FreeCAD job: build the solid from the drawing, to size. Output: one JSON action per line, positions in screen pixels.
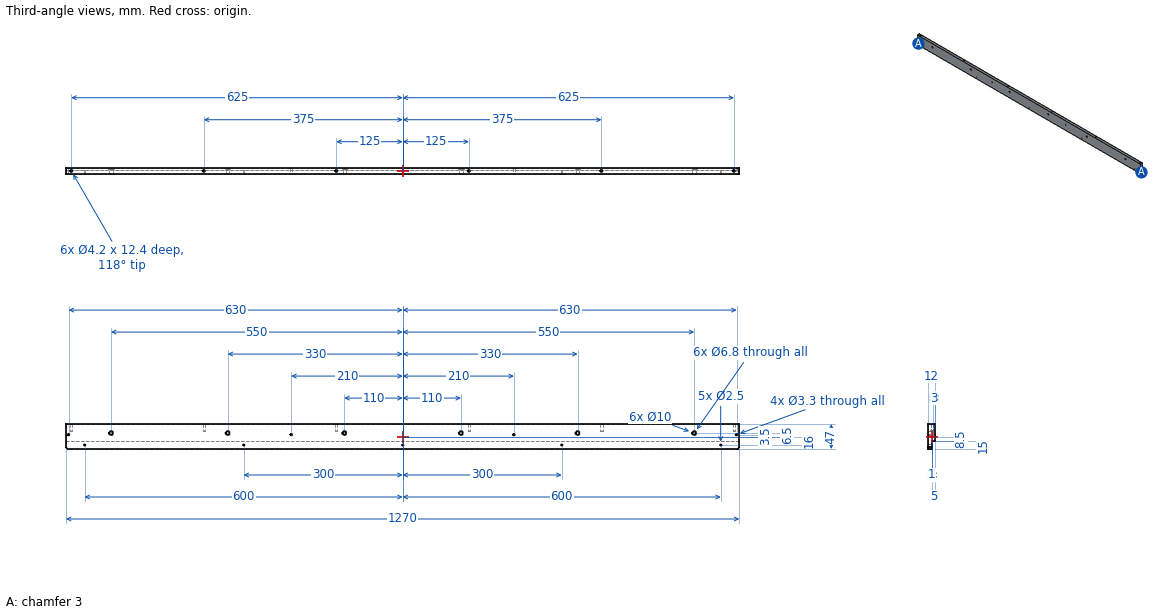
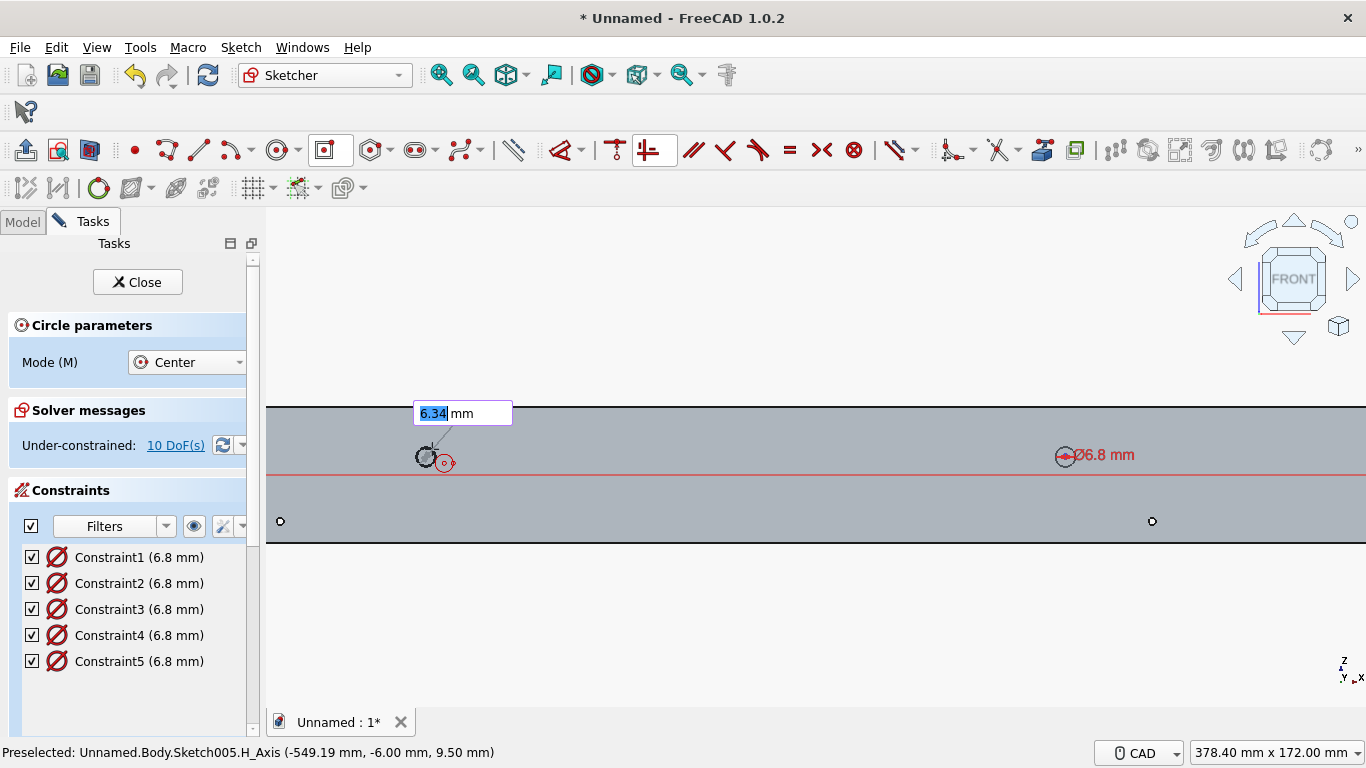
{"action": "type", "text": "6.8"}
{"action": "key", "text": "Return"}
{"action": "key", "text": "Escape"}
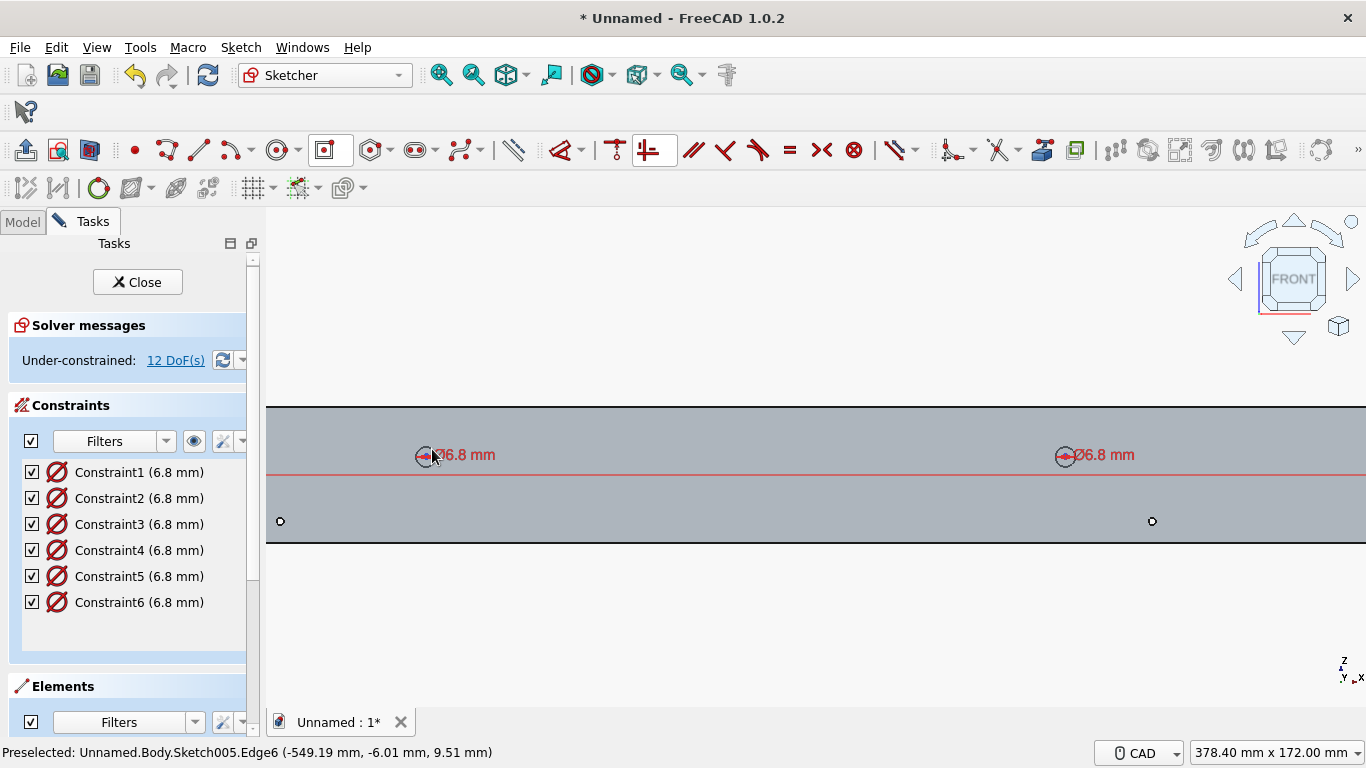
{"action": "scroll", "coordinate": [425, 456], "scroll_direction": "down", "scroll_amount": 8}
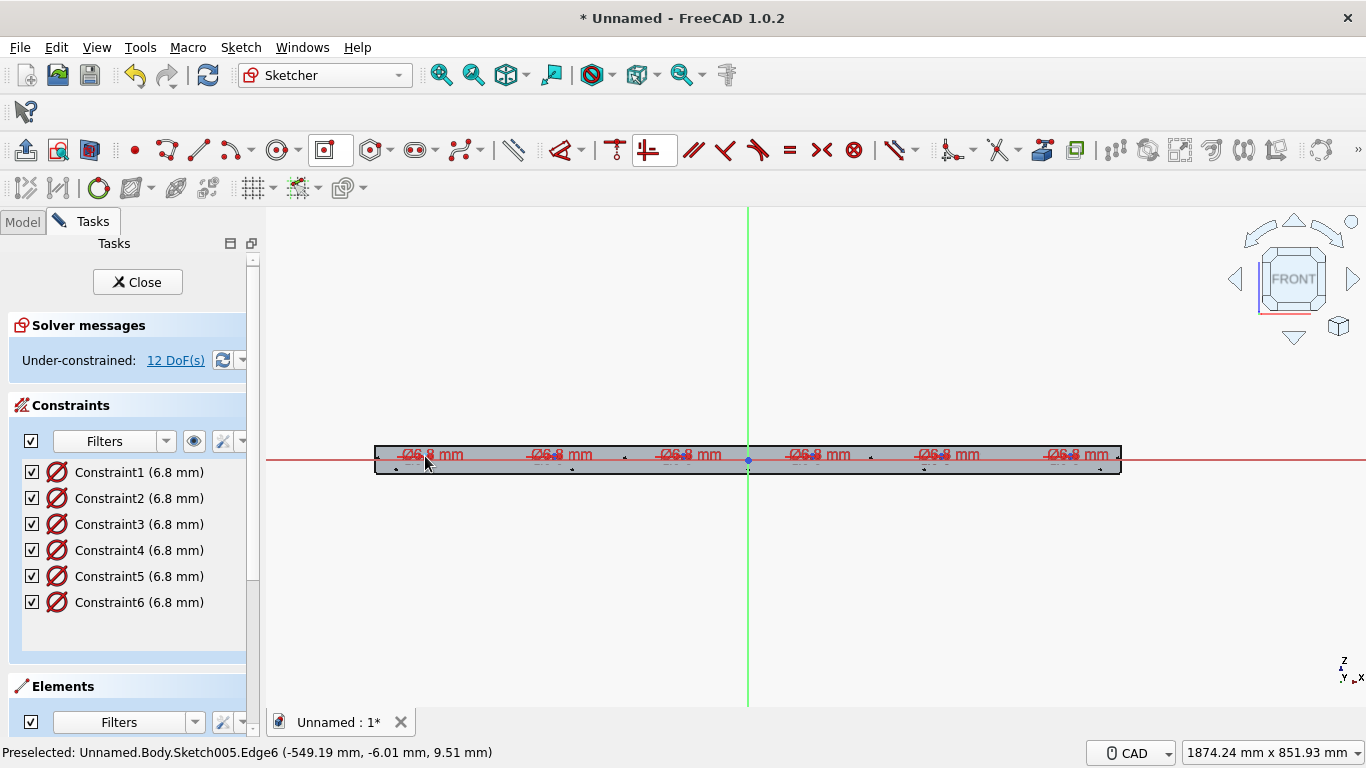
{"action": "left_click", "coordinate": [1071, 457]}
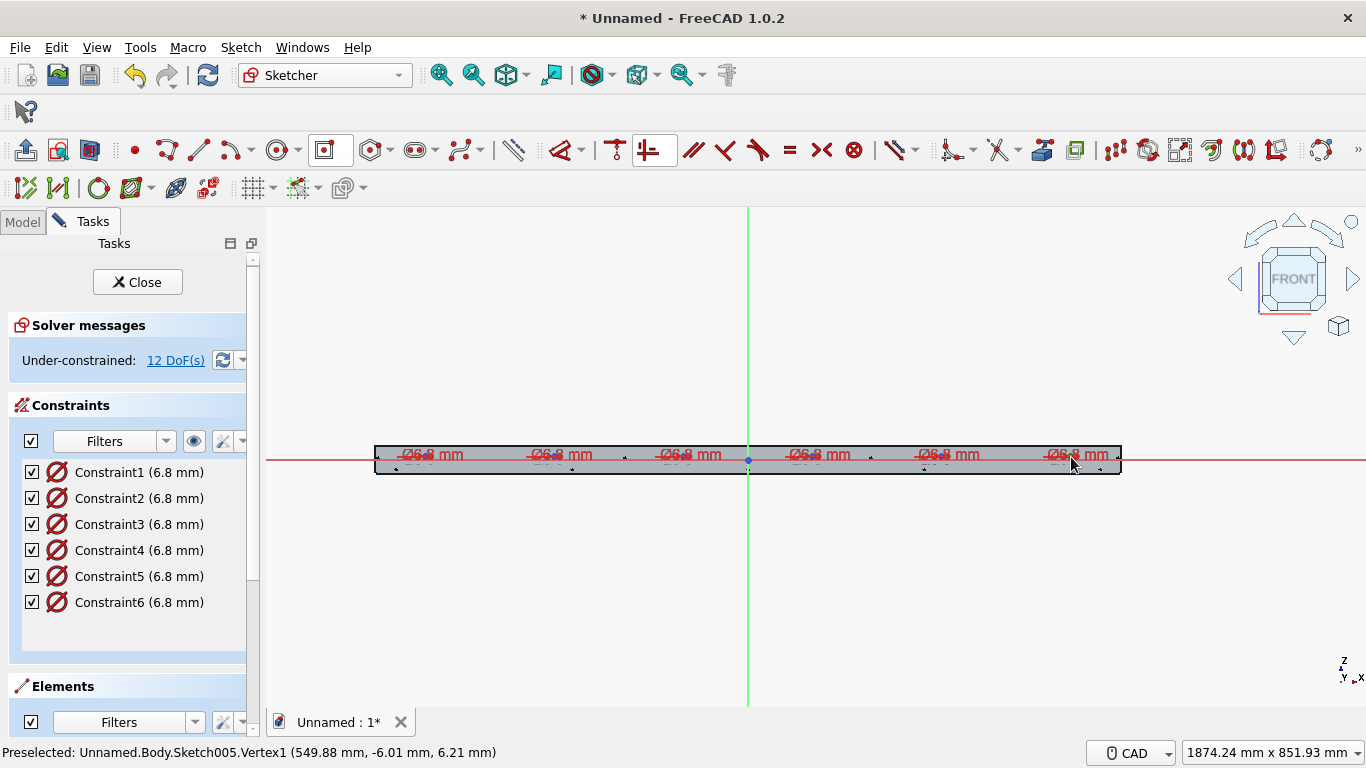
{"action": "left_click", "coordinate": [942, 457]}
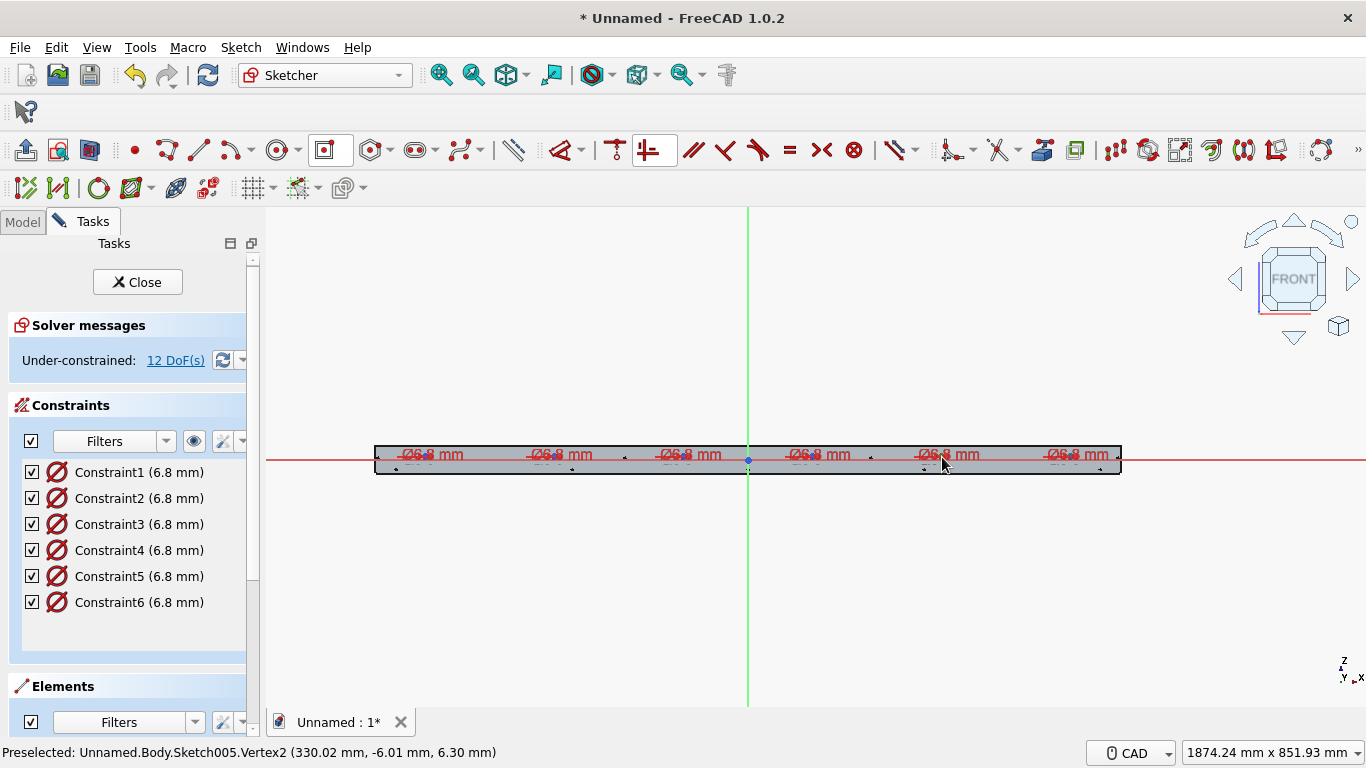
{"action": "key", "text": "h"}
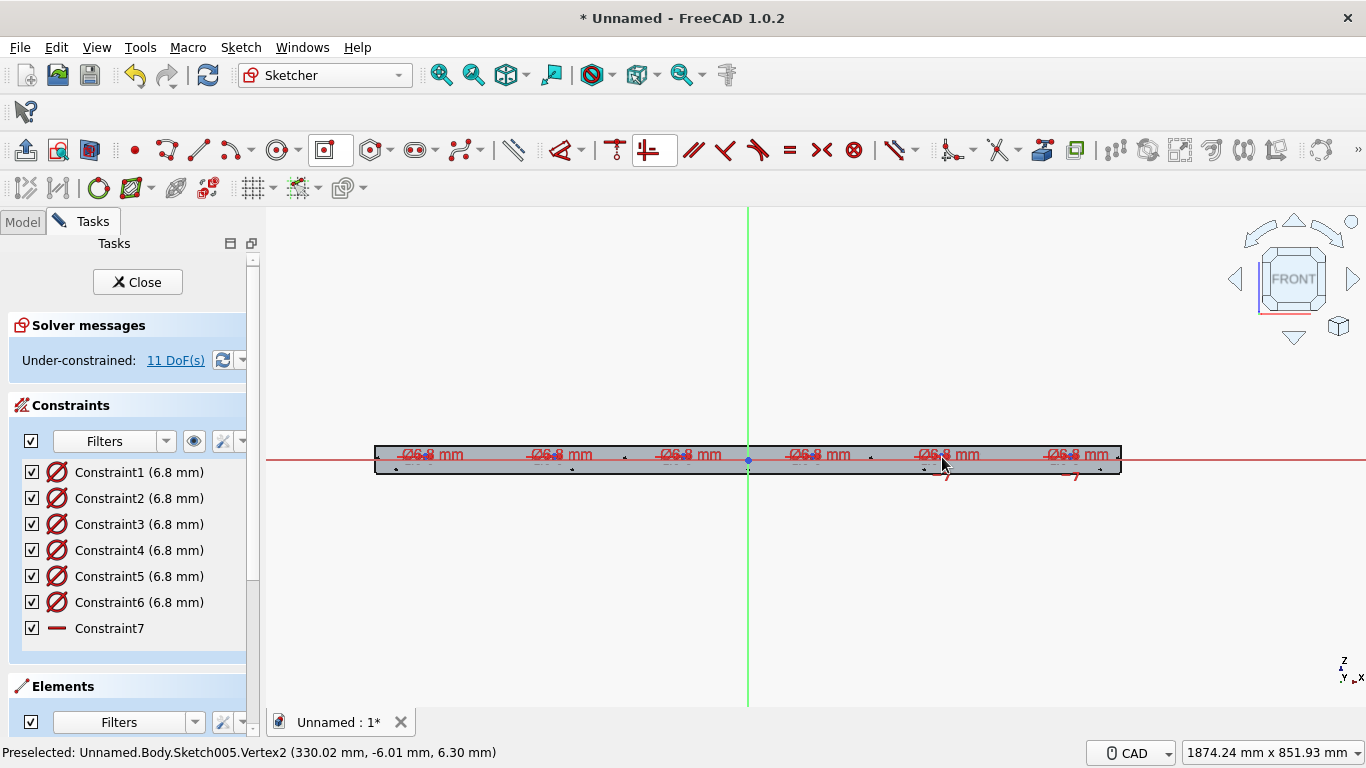
{"action": "left_click", "coordinate": [942, 457]}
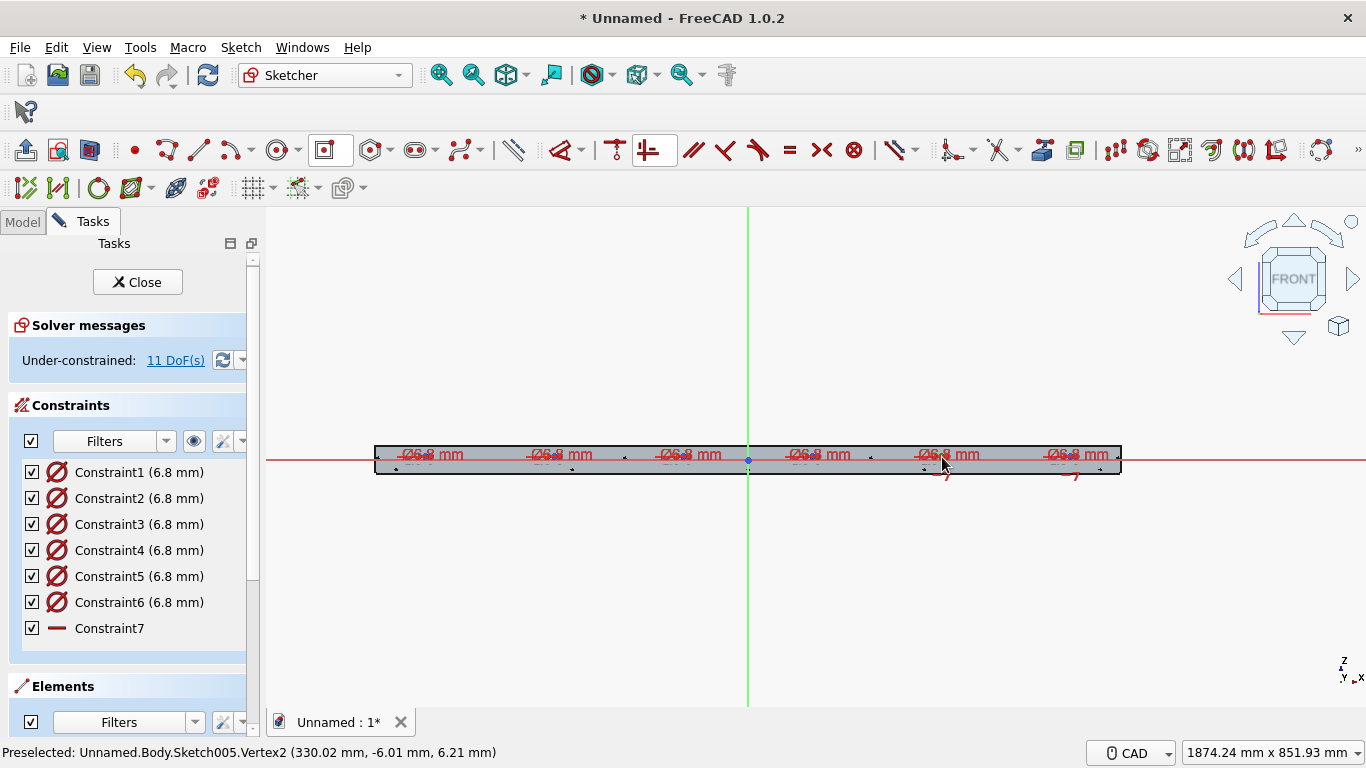
{"action": "left_click", "coordinate": [813, 457]}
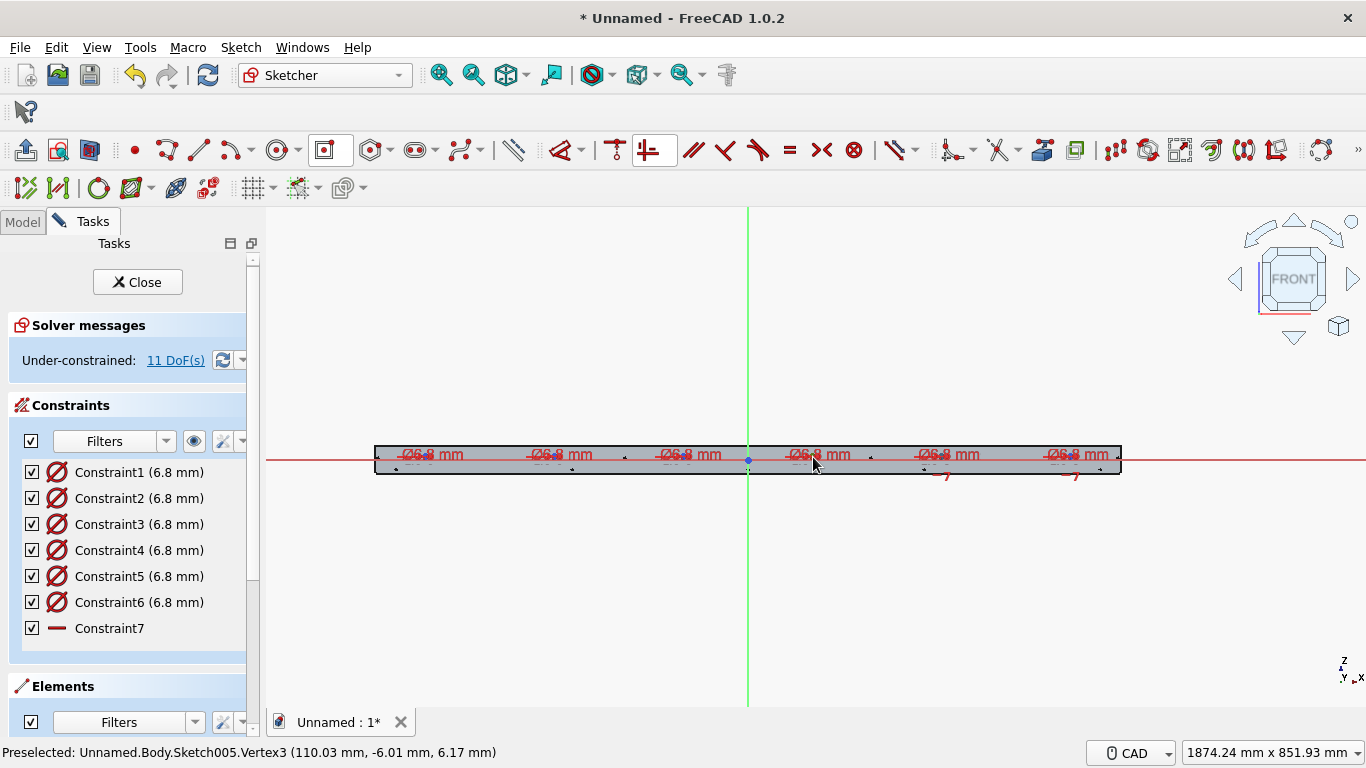
{"action": "left_click", "coordinate": [672, 150]}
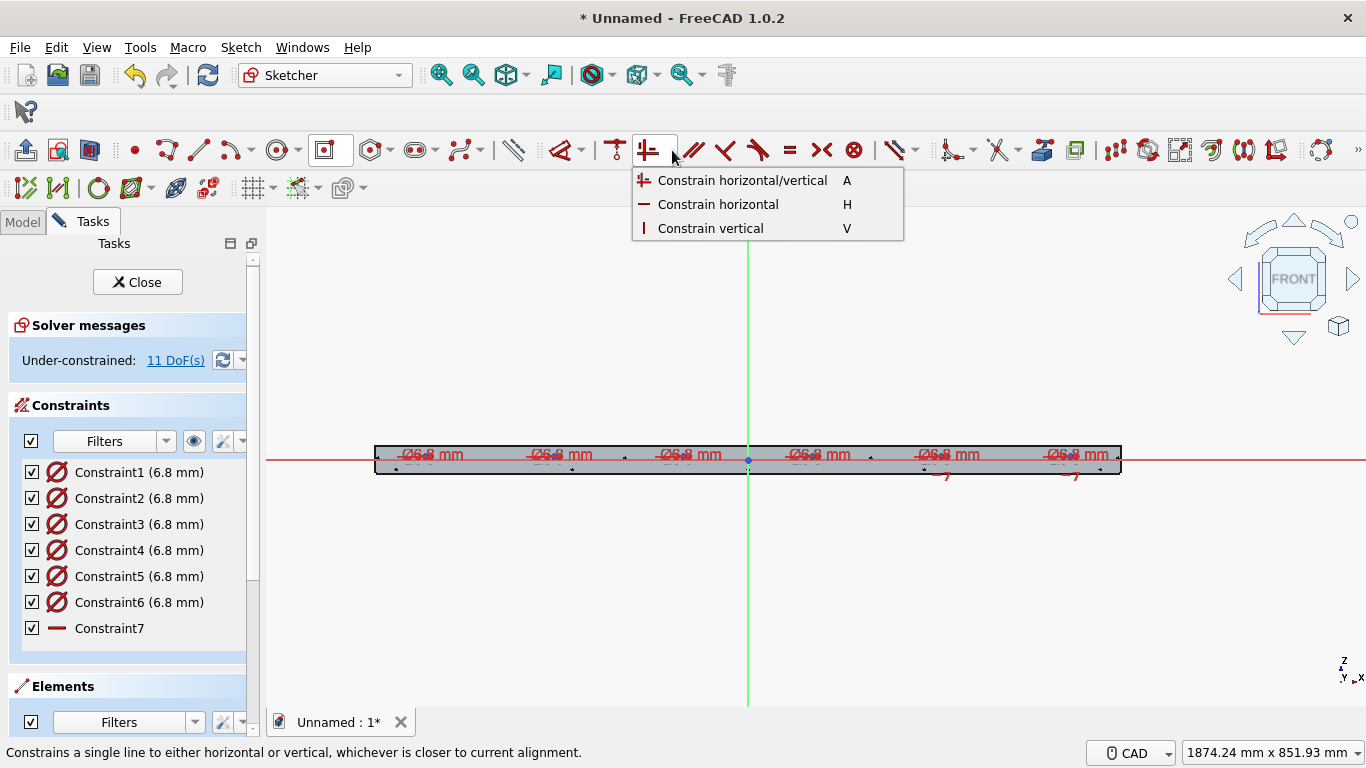
{"action": "left_click", "coordinate": [768, 204]}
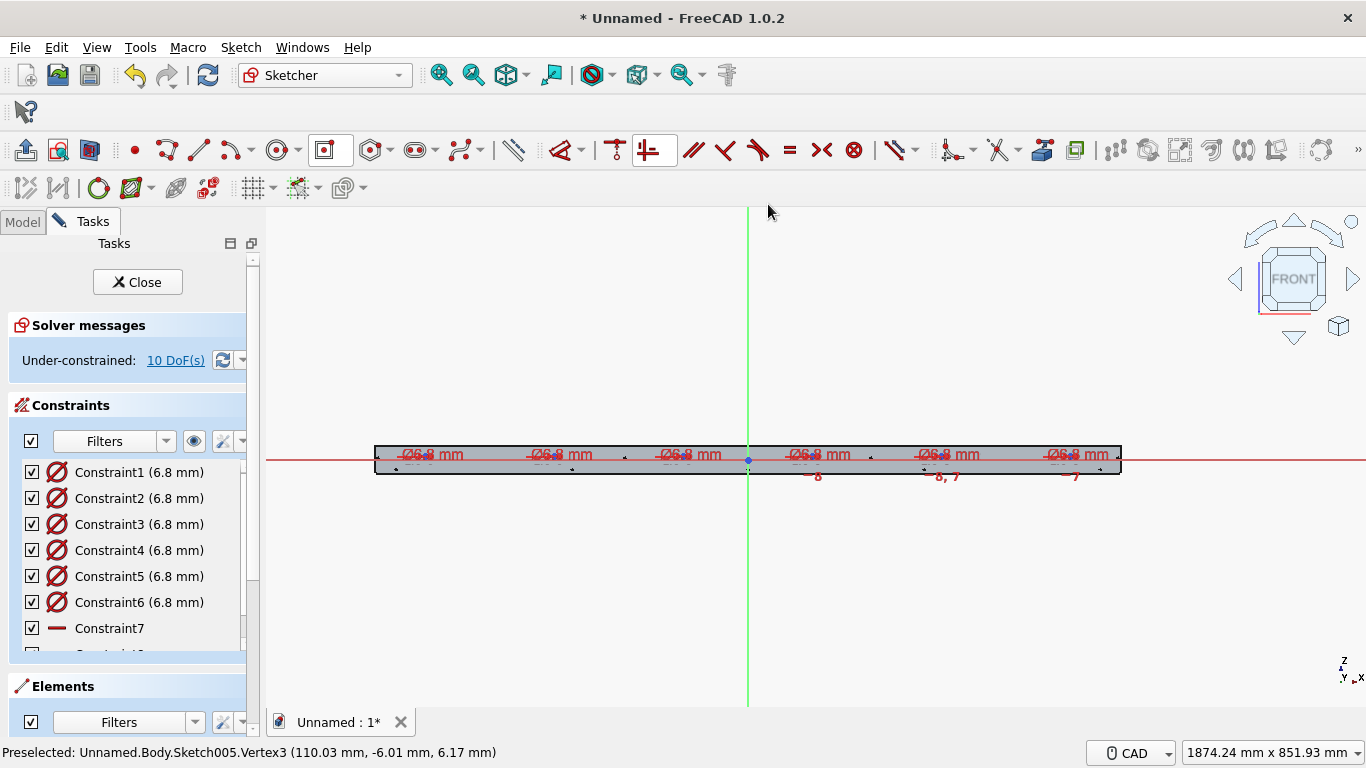
{"action": "left_click", "coordinate": [813, 457]}